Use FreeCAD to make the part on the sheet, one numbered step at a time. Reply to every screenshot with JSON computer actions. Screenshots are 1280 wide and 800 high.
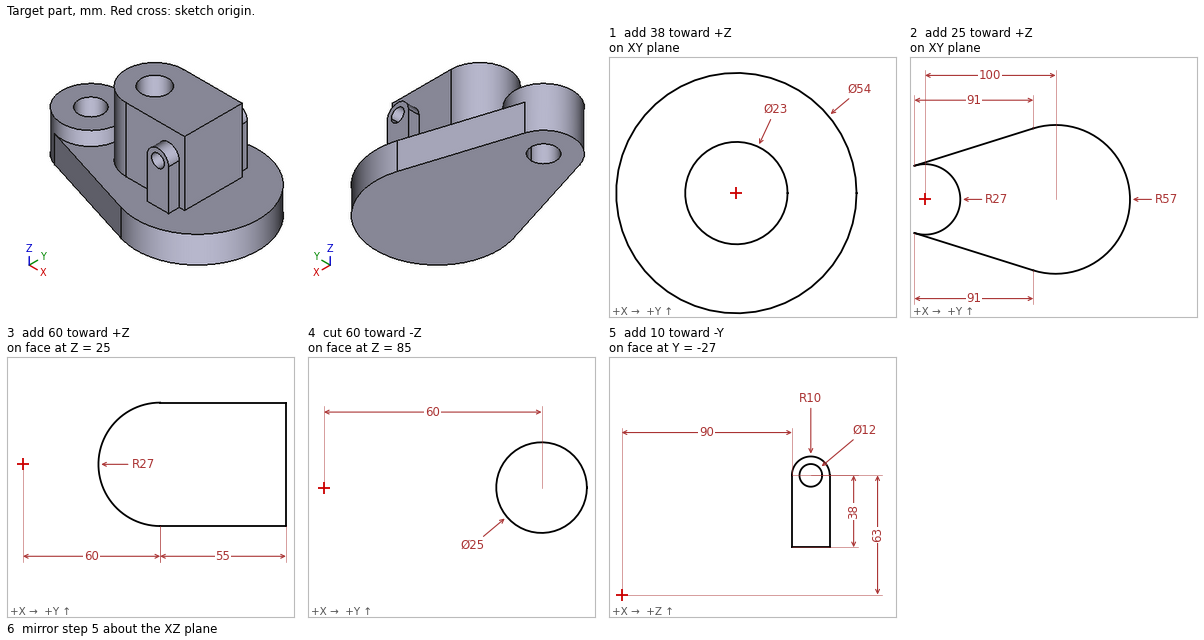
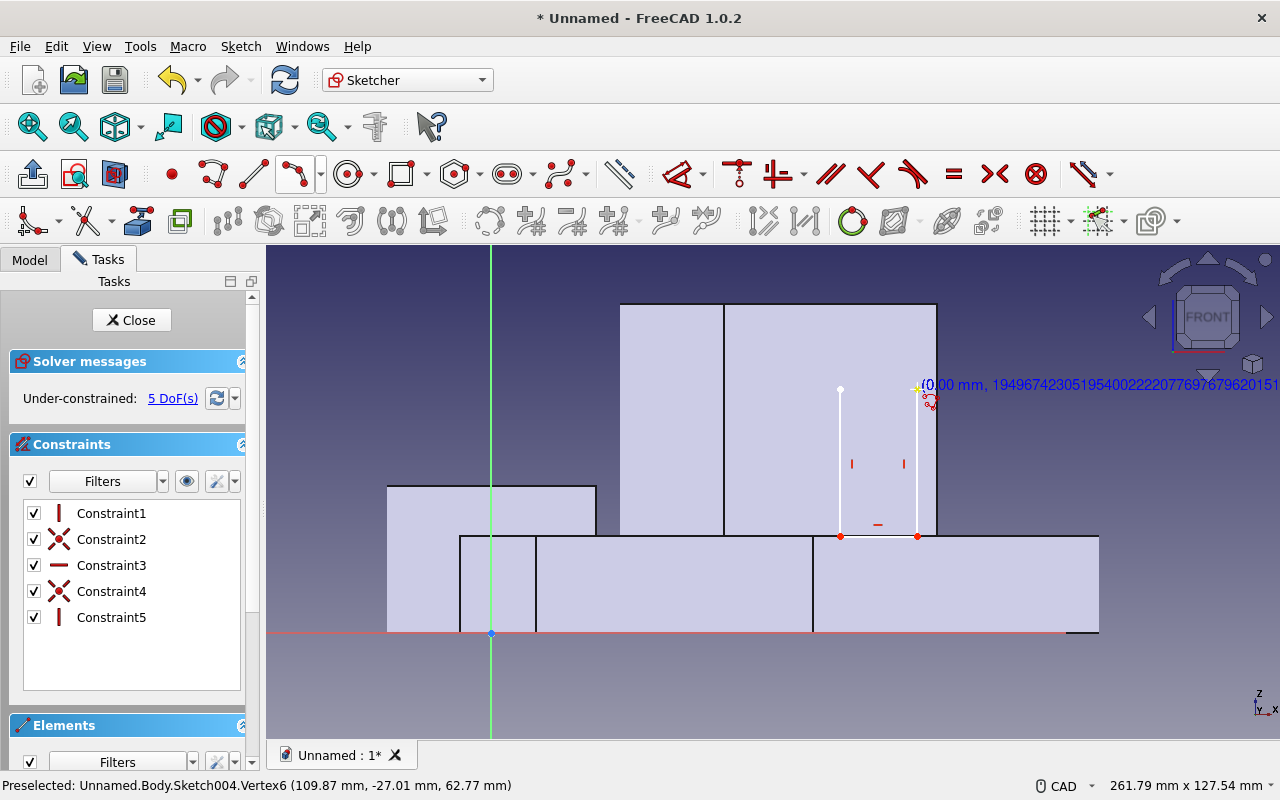
{"action": "key", "text": "g 3 a"}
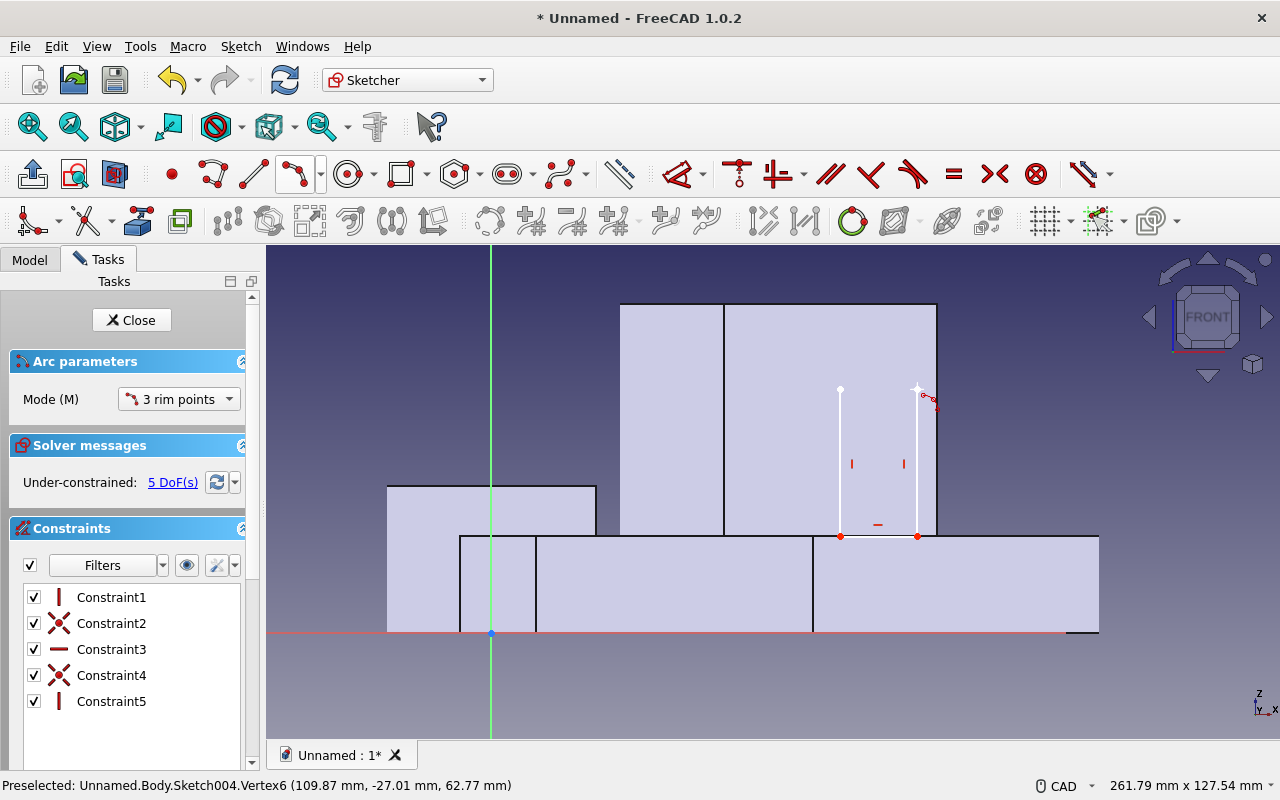
{"action": "left_click", "coordinate": [917, 390]}
{"action": "left_click", "coordinate": [840, 390]}
{"action": "left_click", "coordinate": [879, 350]}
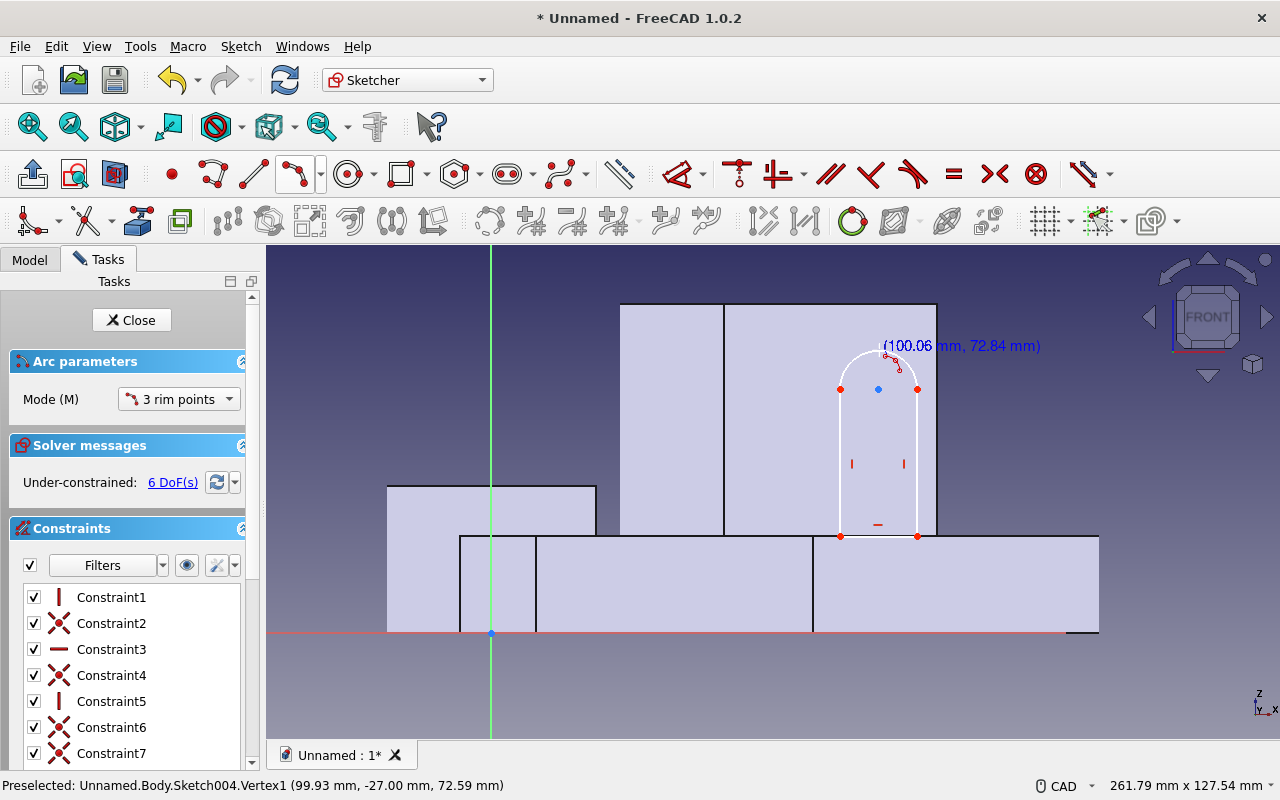
{"action": "key", "text": "g c"}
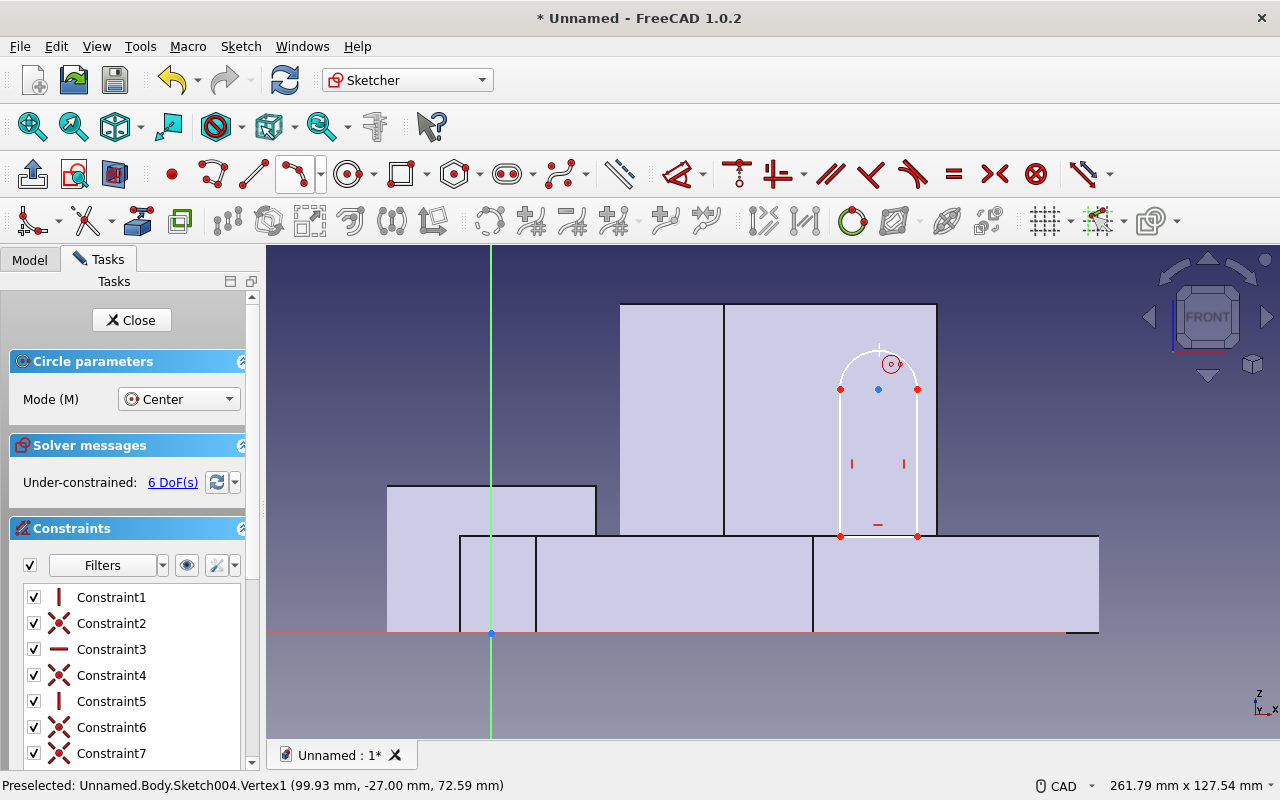
{"action": "left_click", "coordinate": [879, 389]}
{"action": "mouse_move", "coordinate": [895, 373]}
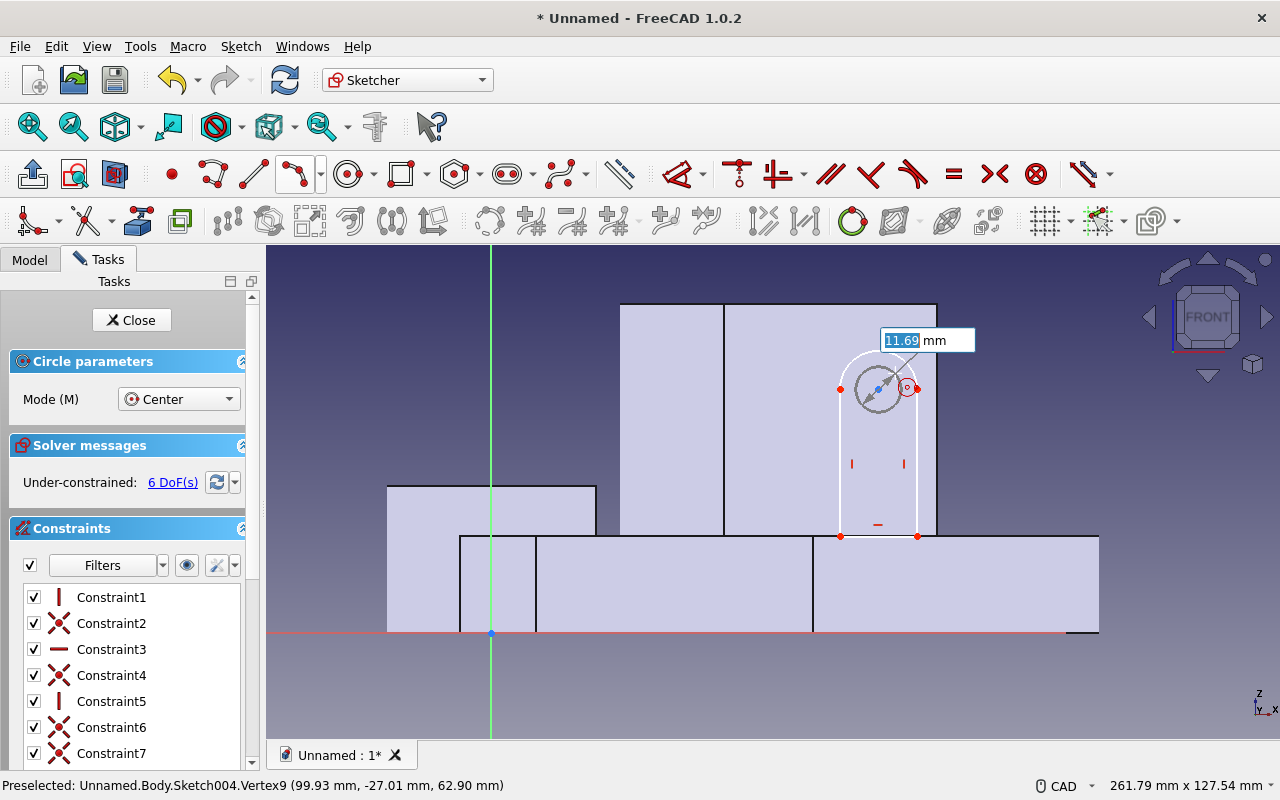
{"action": "type", "text": "12"}
{"action": "key", "text": "Return"}
{"action": "key", "text": "Escape"}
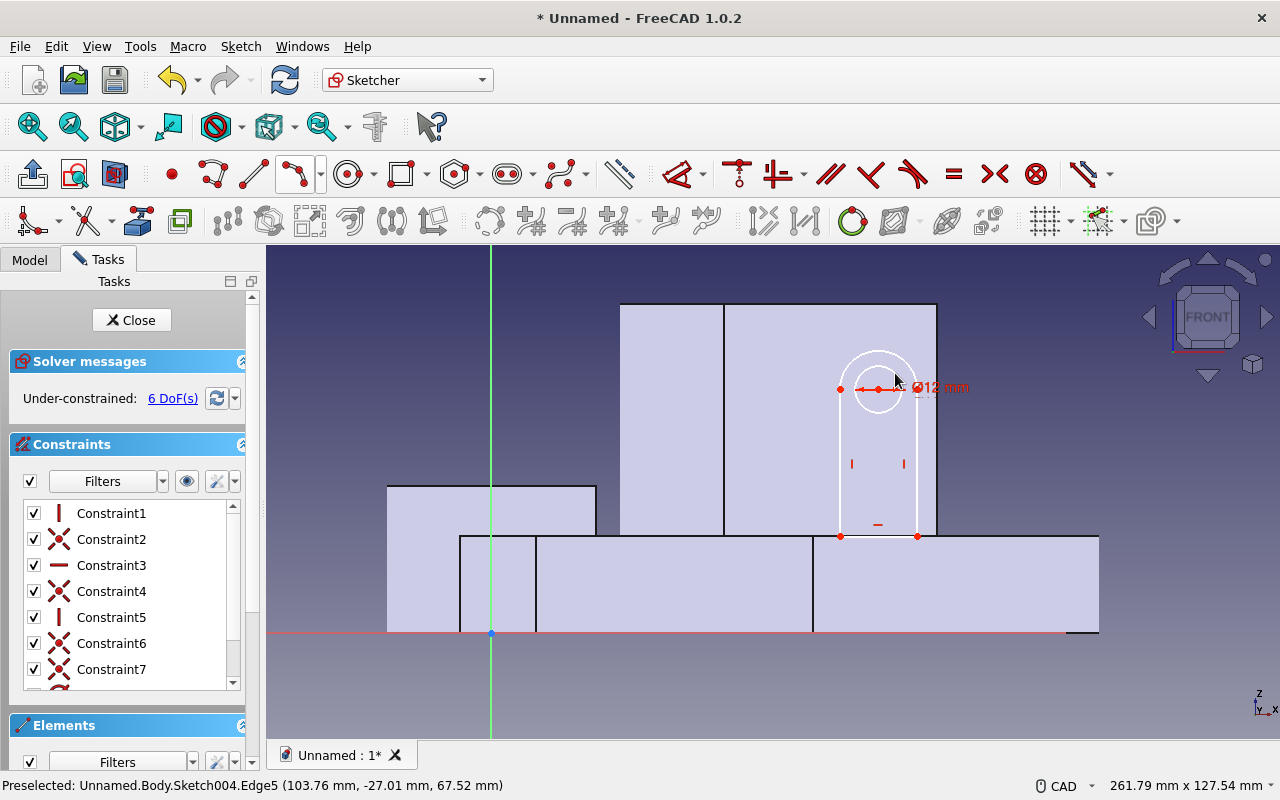
{"action": "left_click", "coordinate": [840, 434]}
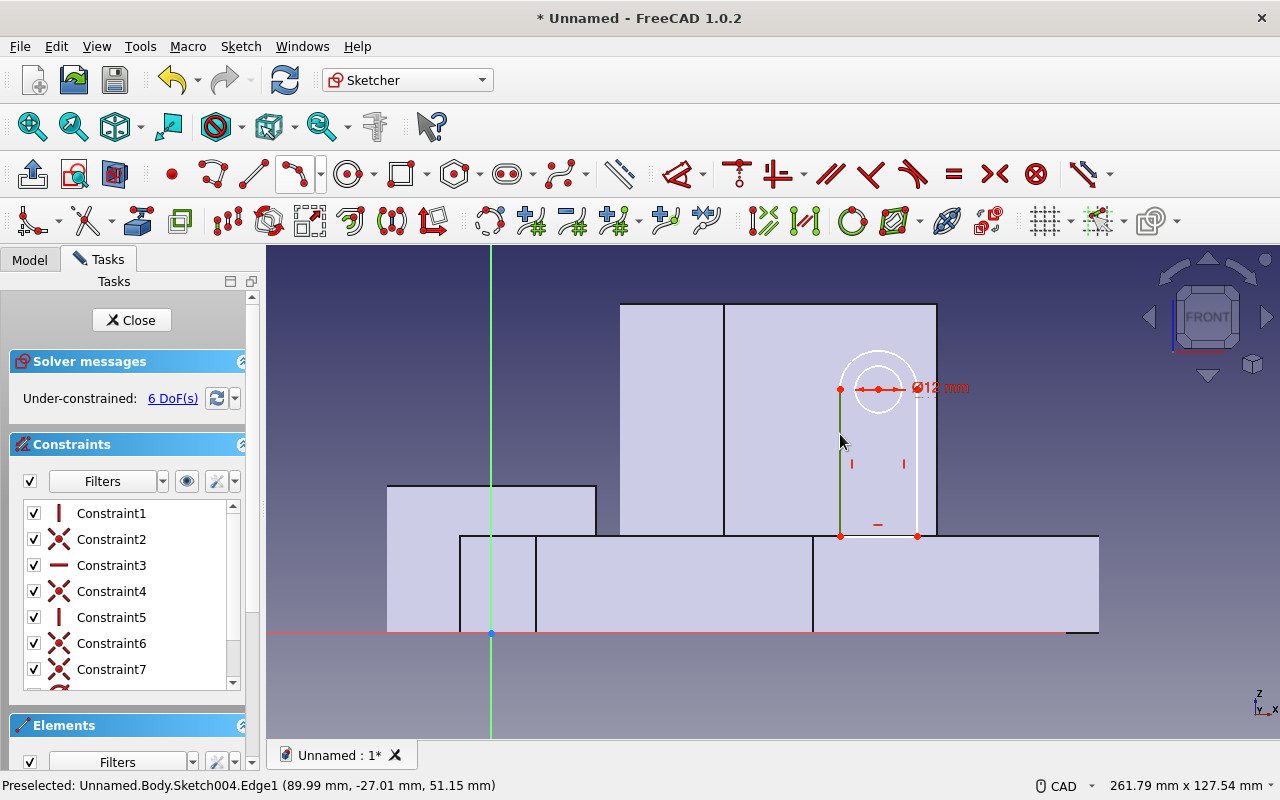
{"action": "left_click", "coordinate": [901, 358]}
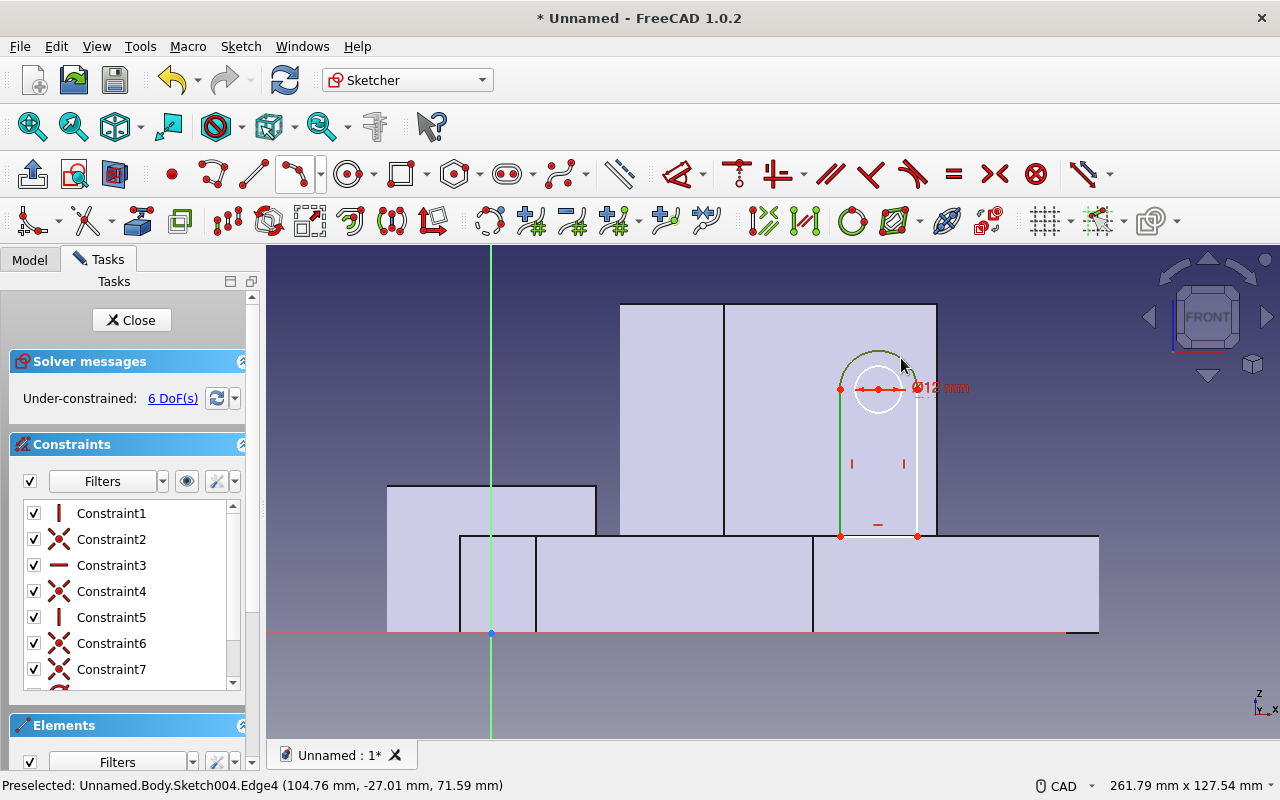
{"action": "key", "text": "t"}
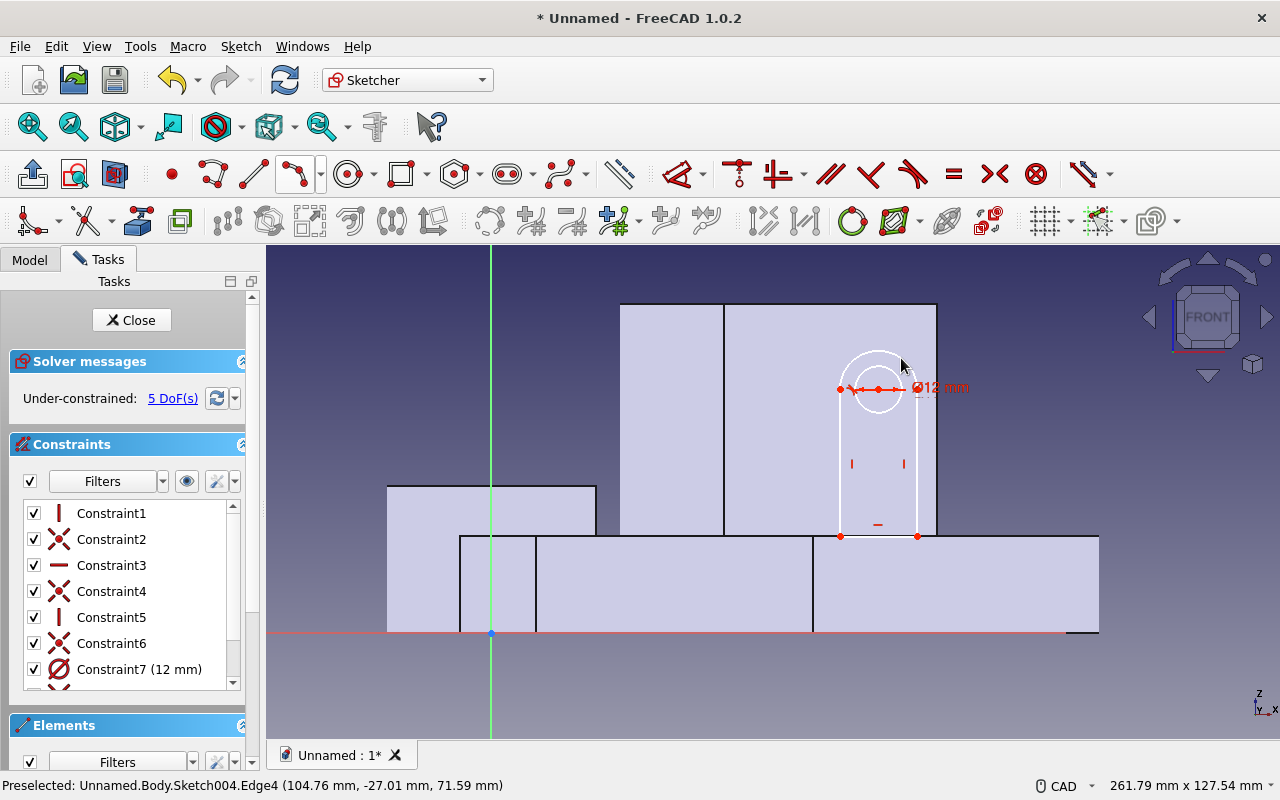
{"action": "left_click", "coordinate": [917, 493]}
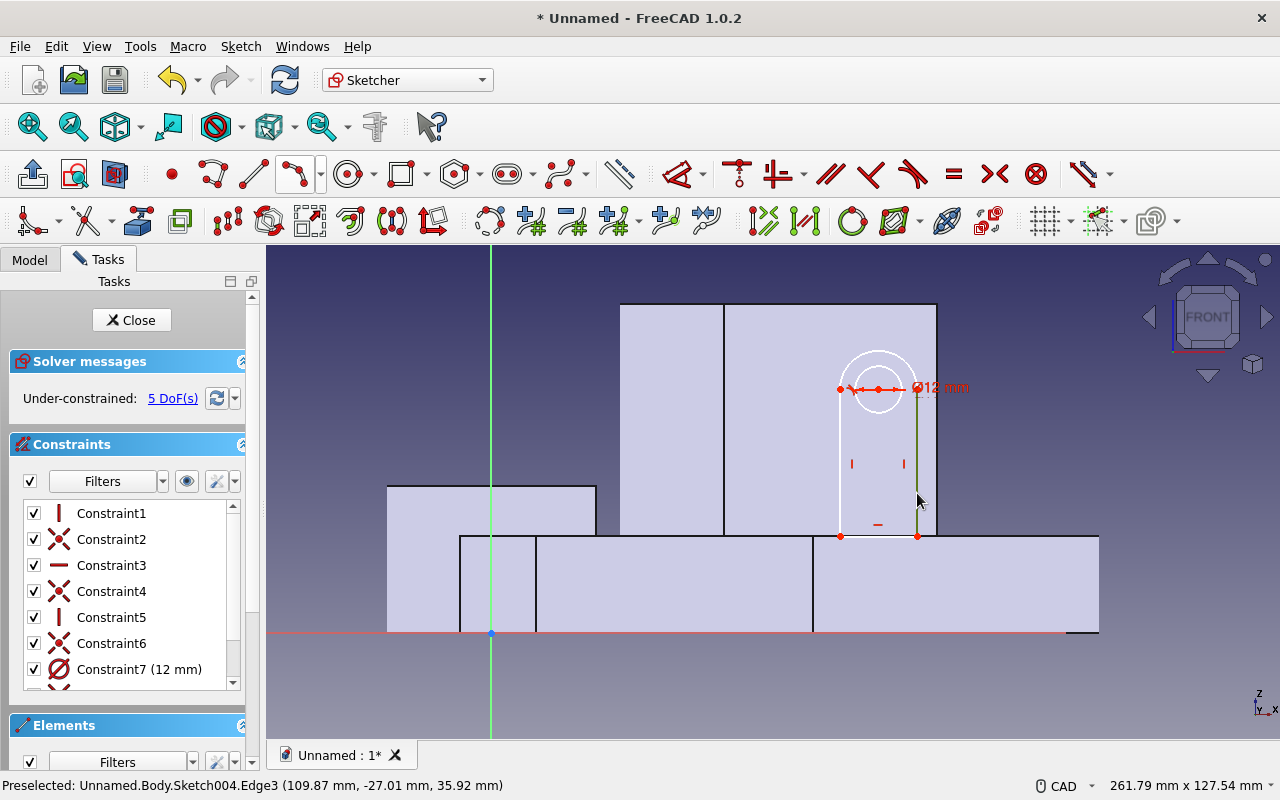
{"action": "left_click", "coordinate": [901, 359]}